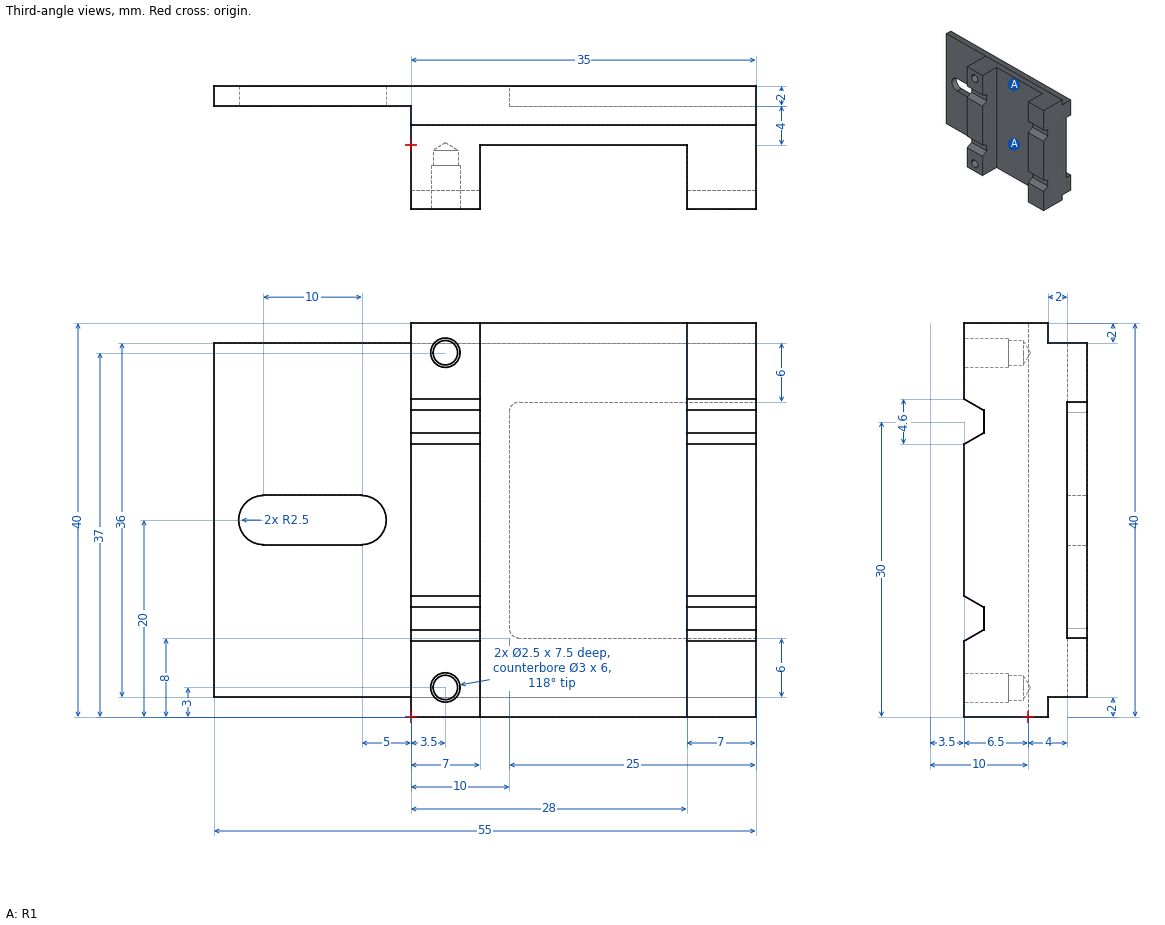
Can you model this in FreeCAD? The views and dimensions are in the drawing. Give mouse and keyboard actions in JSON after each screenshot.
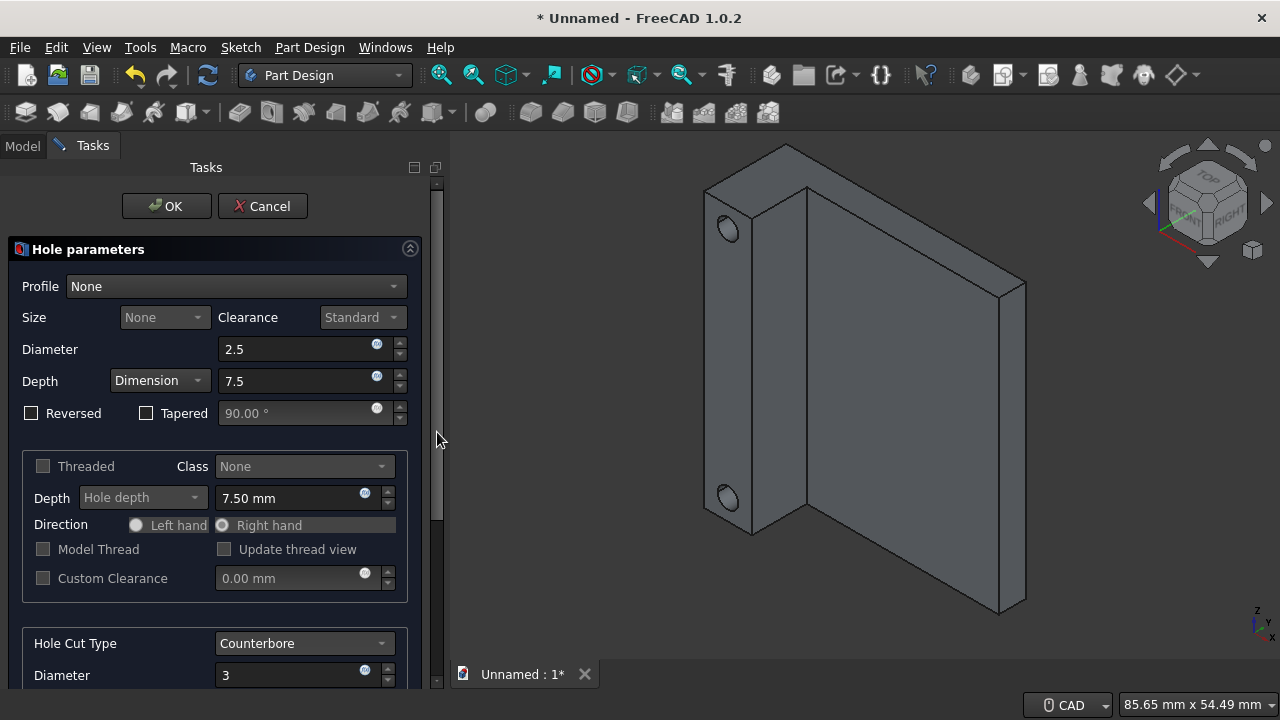
{"action": "left_click", "coordinate": [167, 206]}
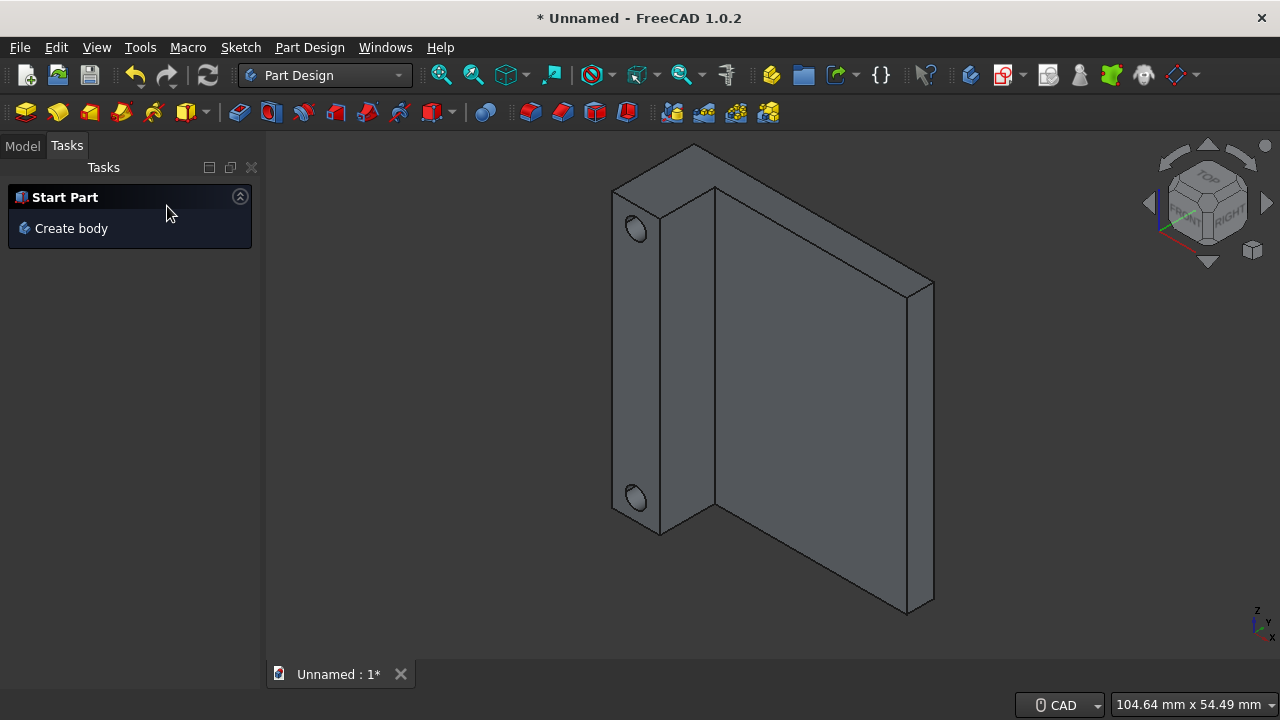
{"action": "left_click", "coordinate": [811, 355]}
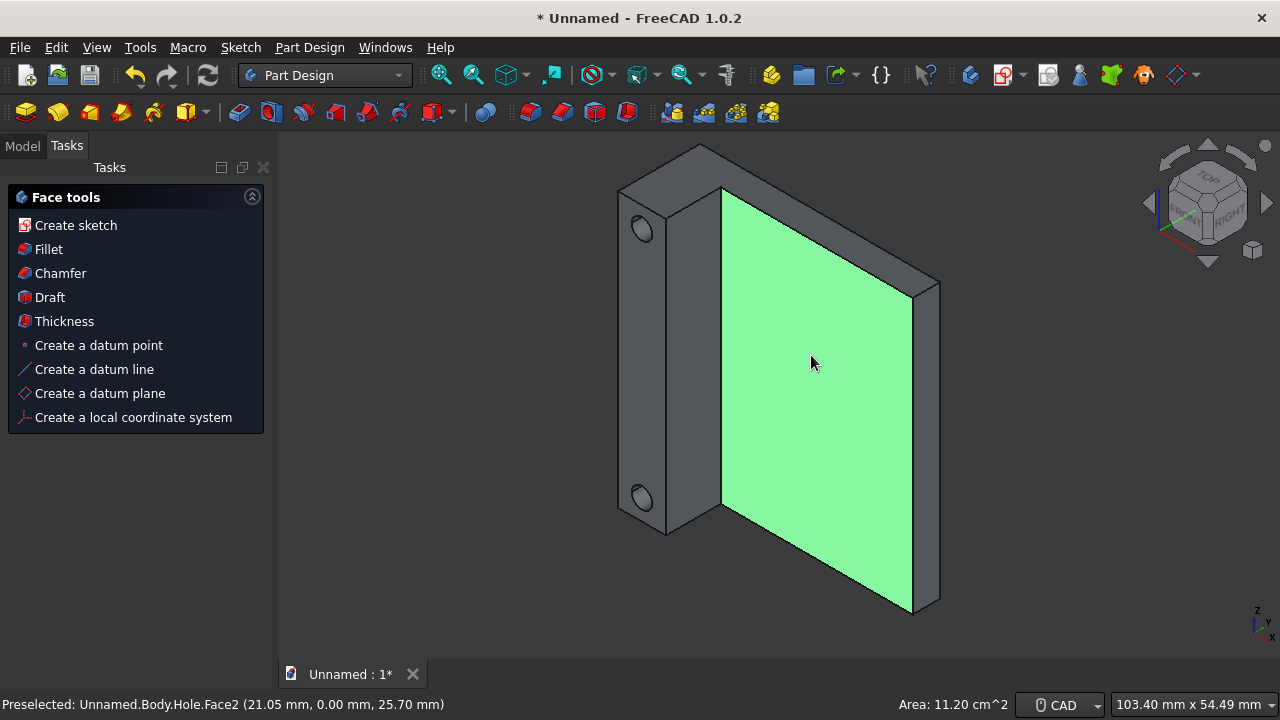
{"action": "left_click", "coordinate": [1004, 76]}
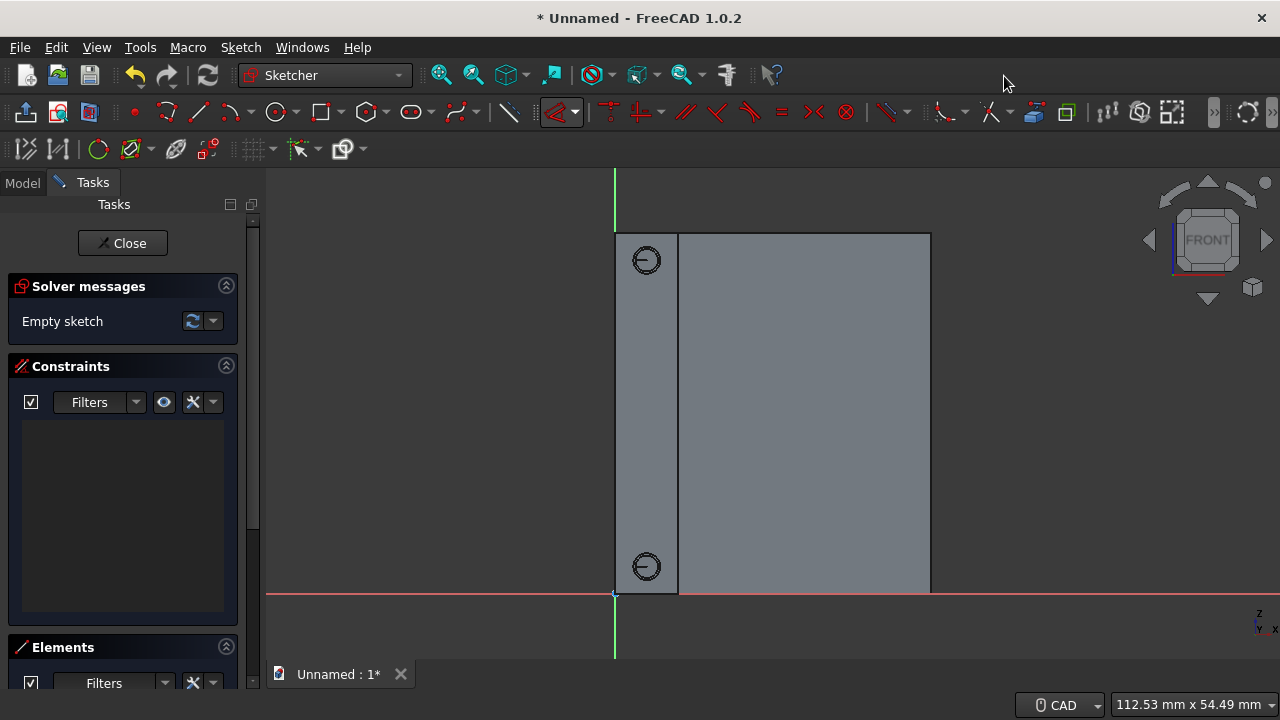
{"action": "left_click", "coordinate": [90, 112]}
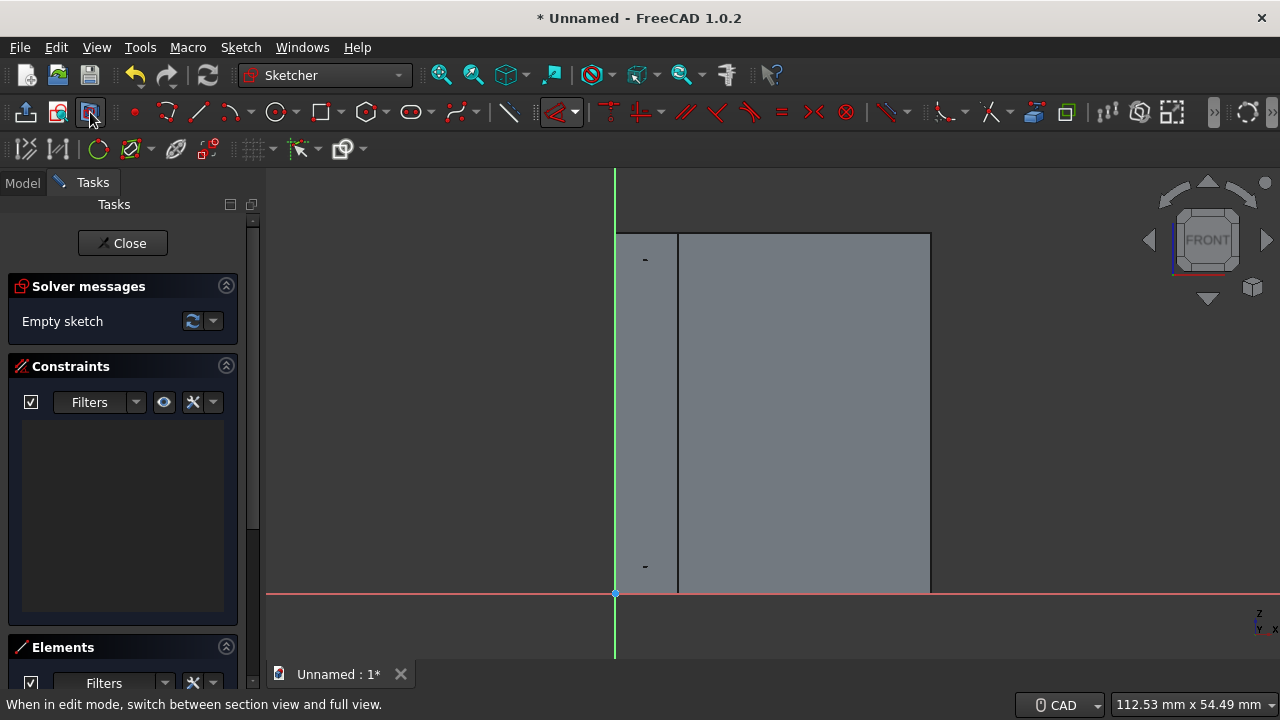
{"action": "left_click", "coordinate": [322, 112]}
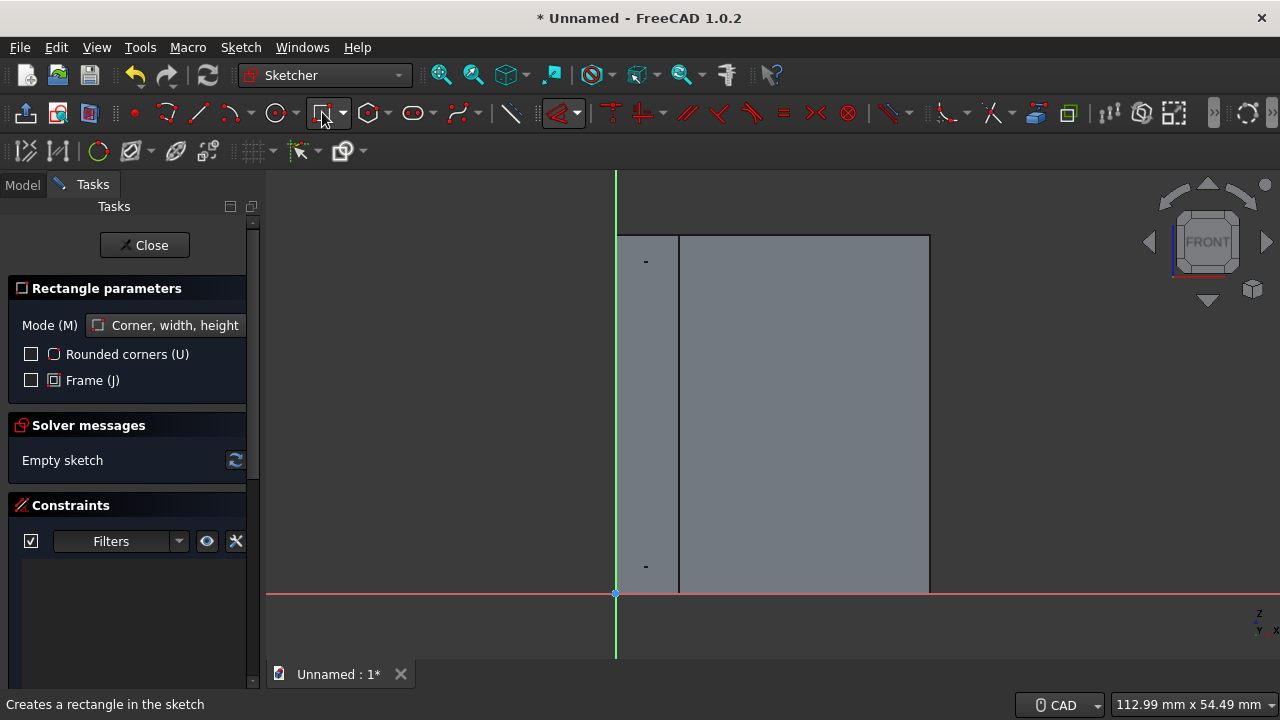
{"action": "left_click", "coordinate": [867, 235]}
{"action": "left_click", "coordinate": [930, 594]}
{"action": "key", "text": "Escape"}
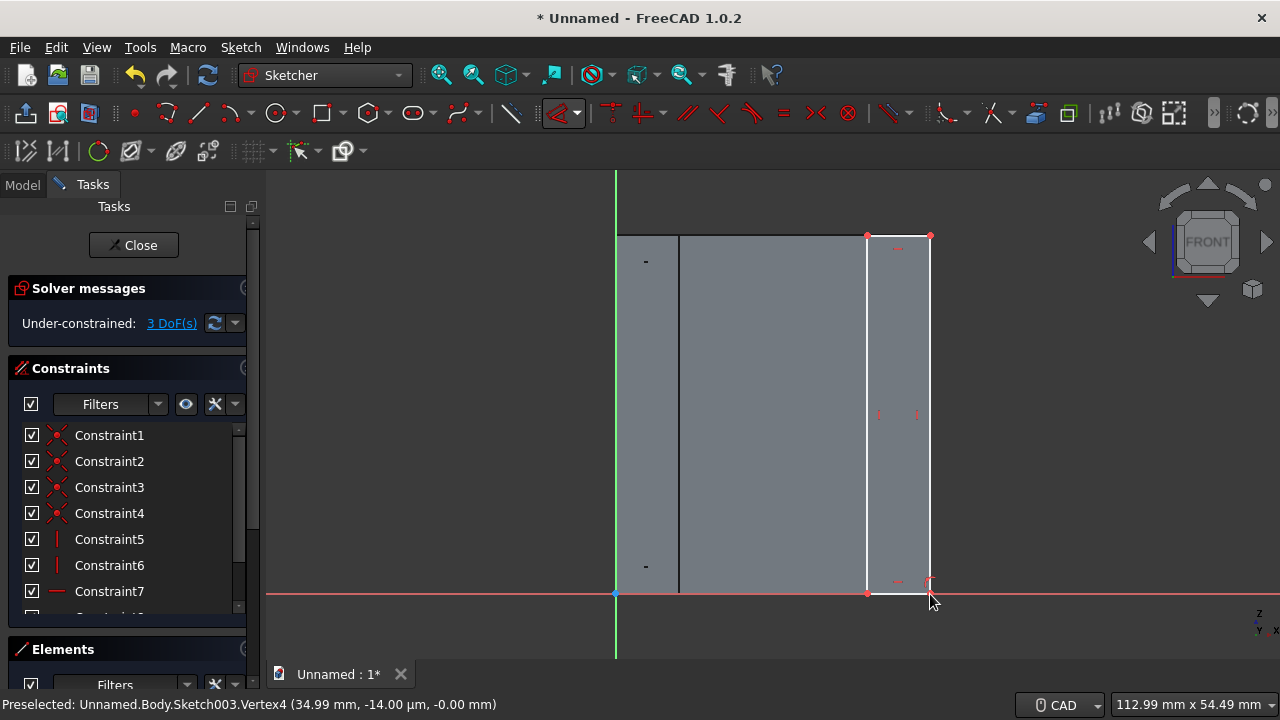
{"action": "left_click", "coordinate": [886, 594]}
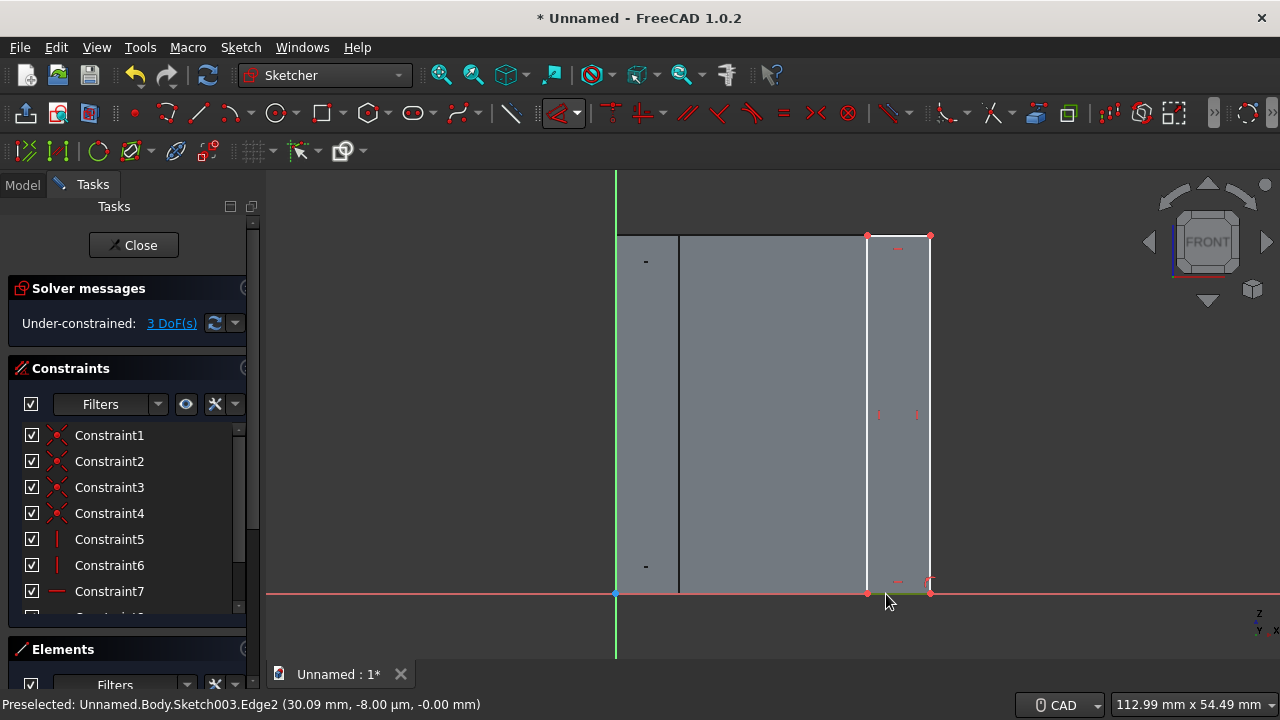
{"action": "key", "text": "l"}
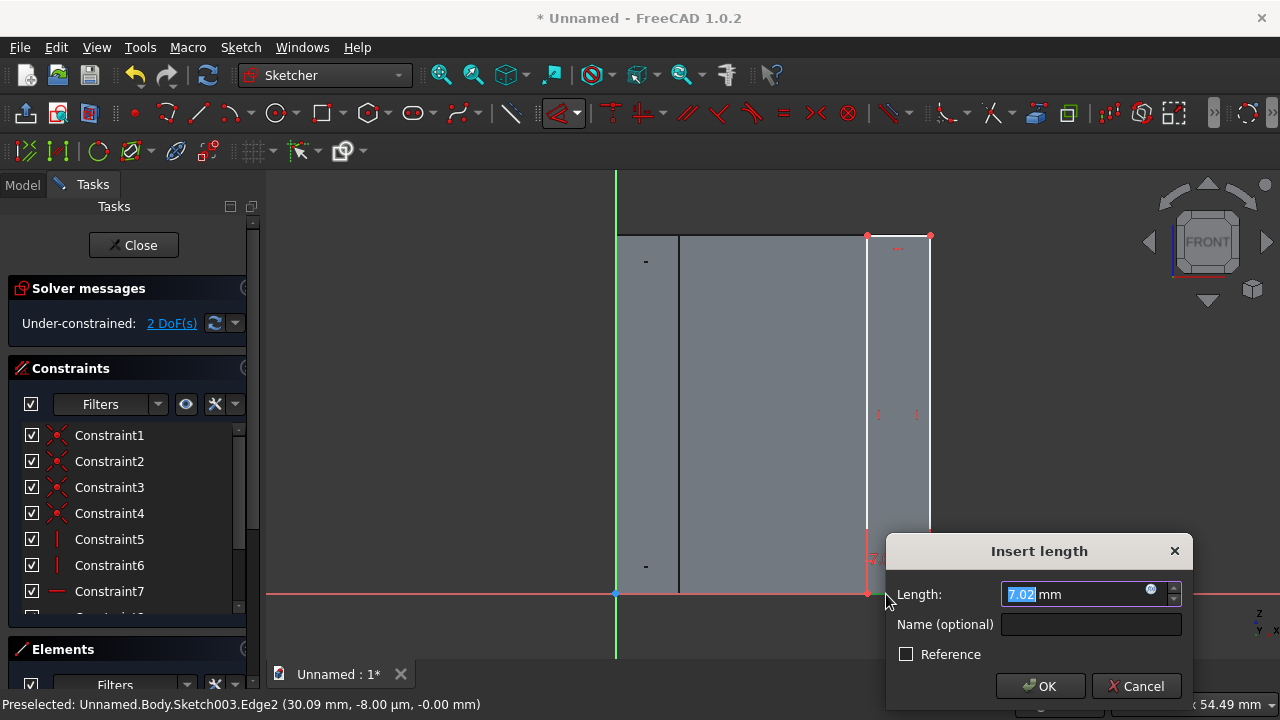
{"action": "type", "text": "7"}
{"action": "key", "text": "Return"}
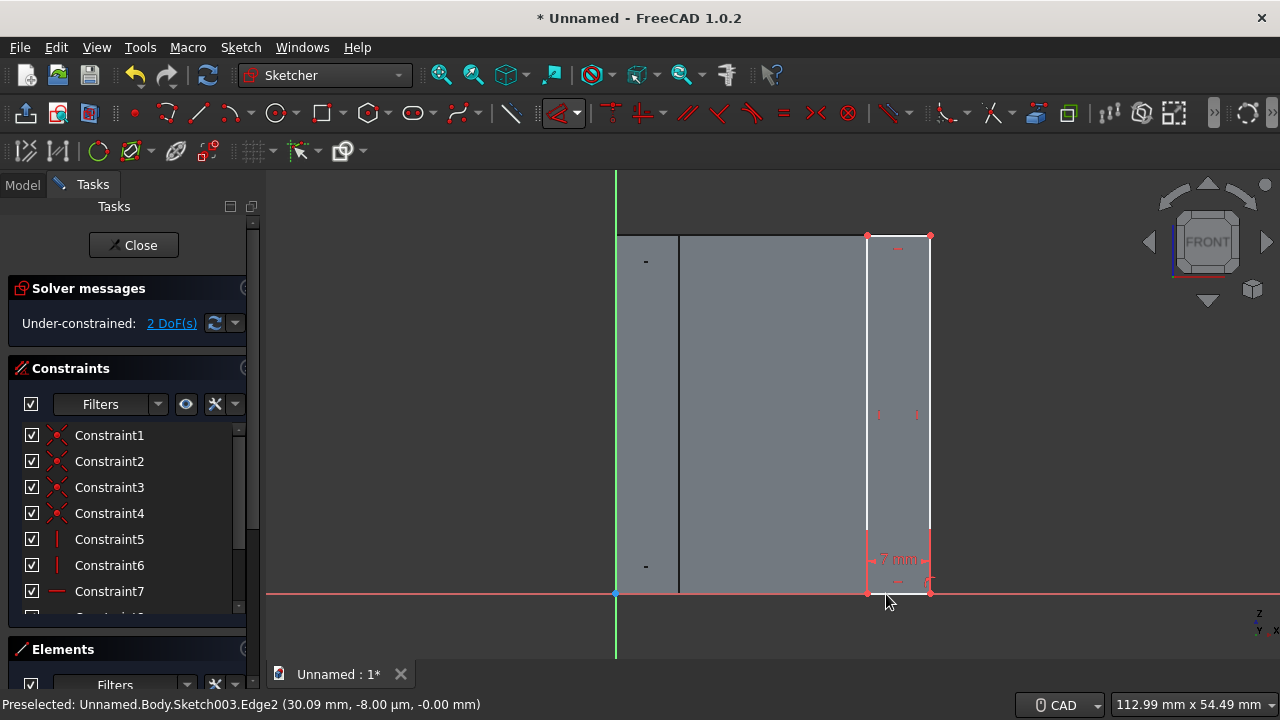
{"action": "left_click", "coordinate": [867, 343]}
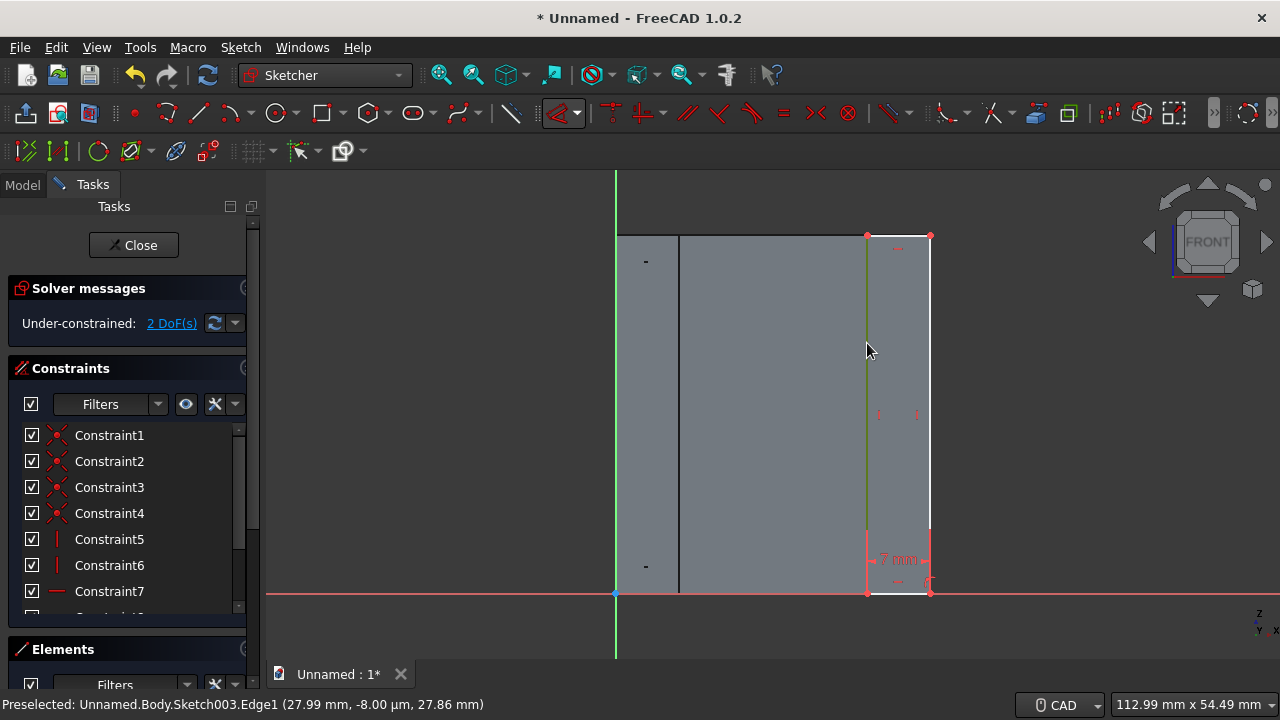
{"action": "left_click", "coordinate": [580, 114]}